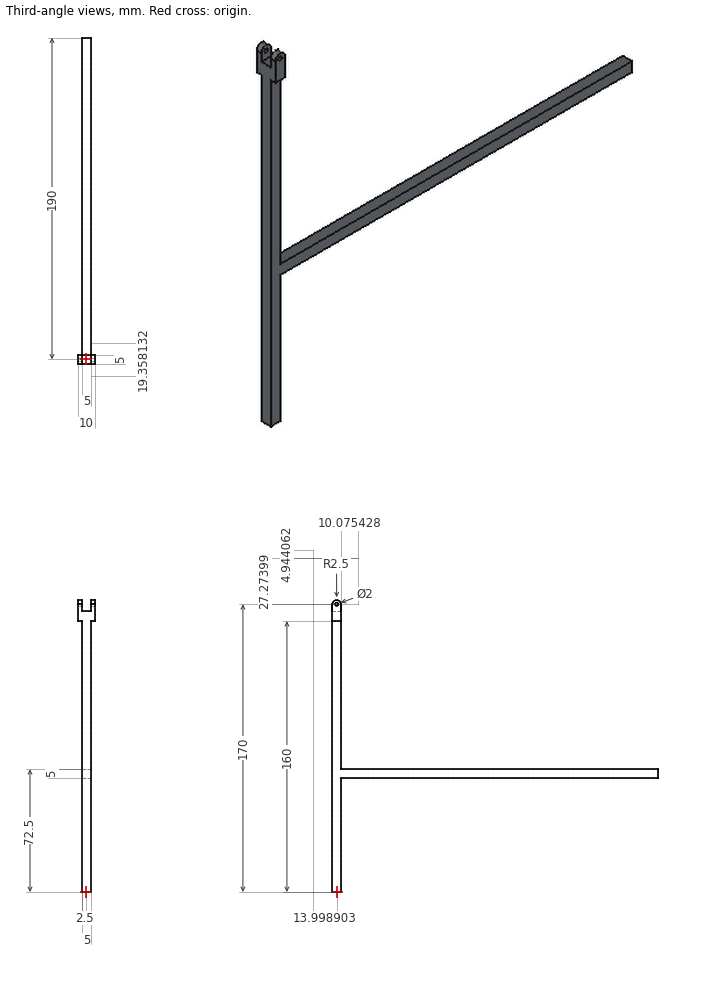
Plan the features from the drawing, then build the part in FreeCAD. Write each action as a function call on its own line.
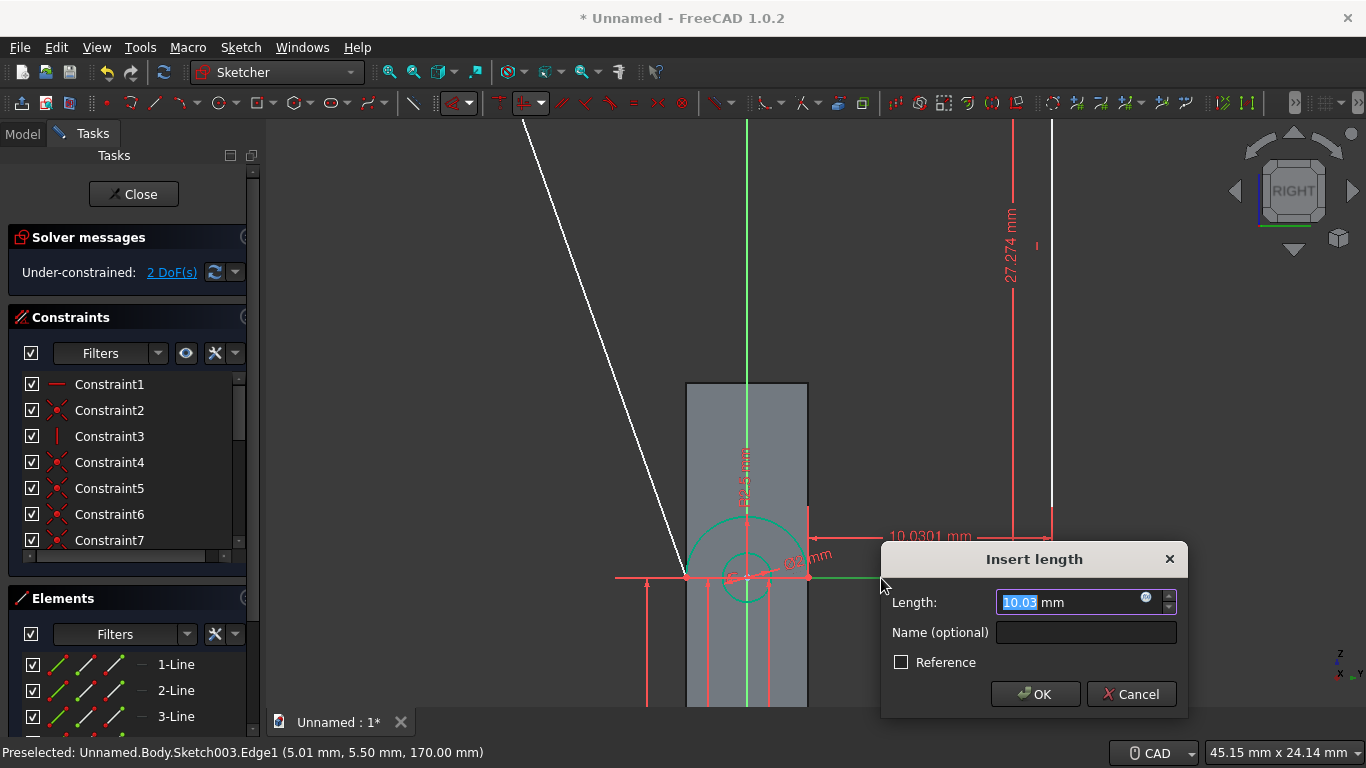
text(10.075428)
key(Return)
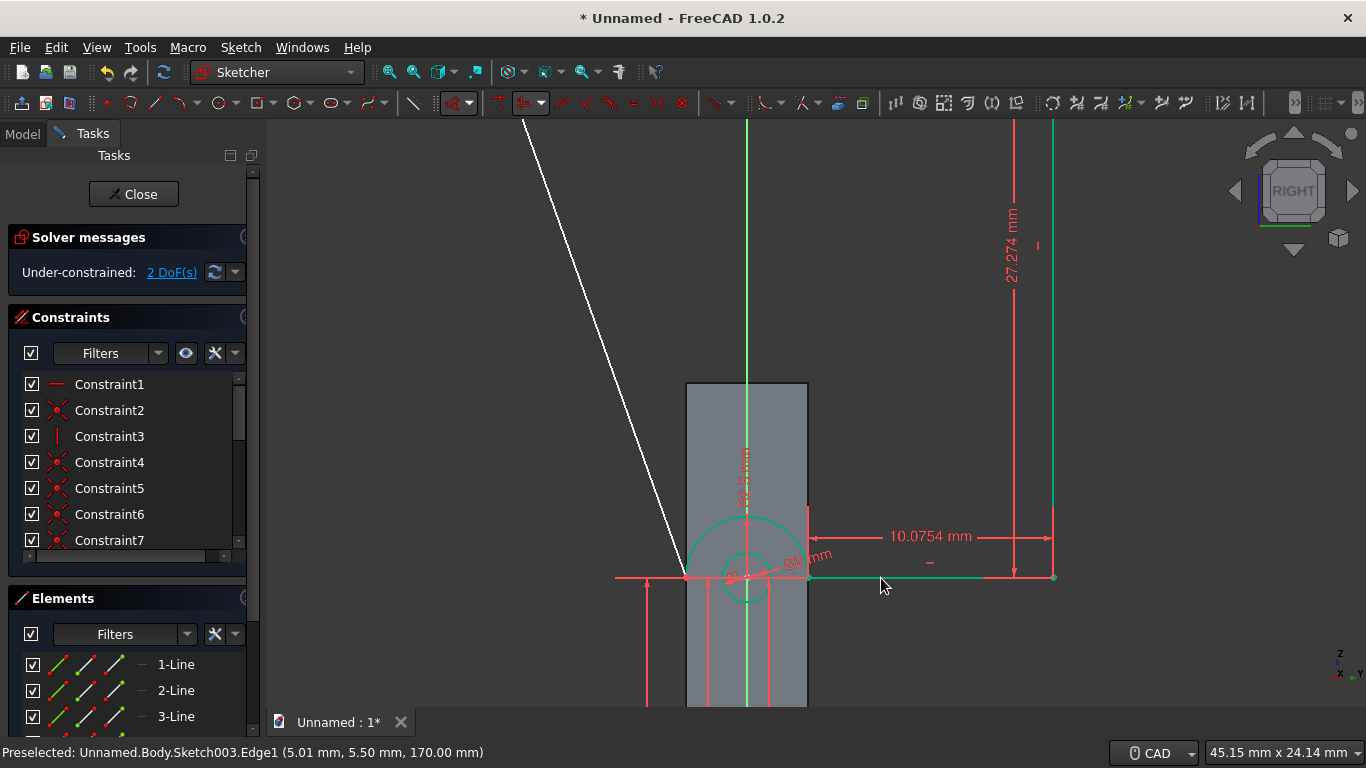
scroll(762, 589, down, 4)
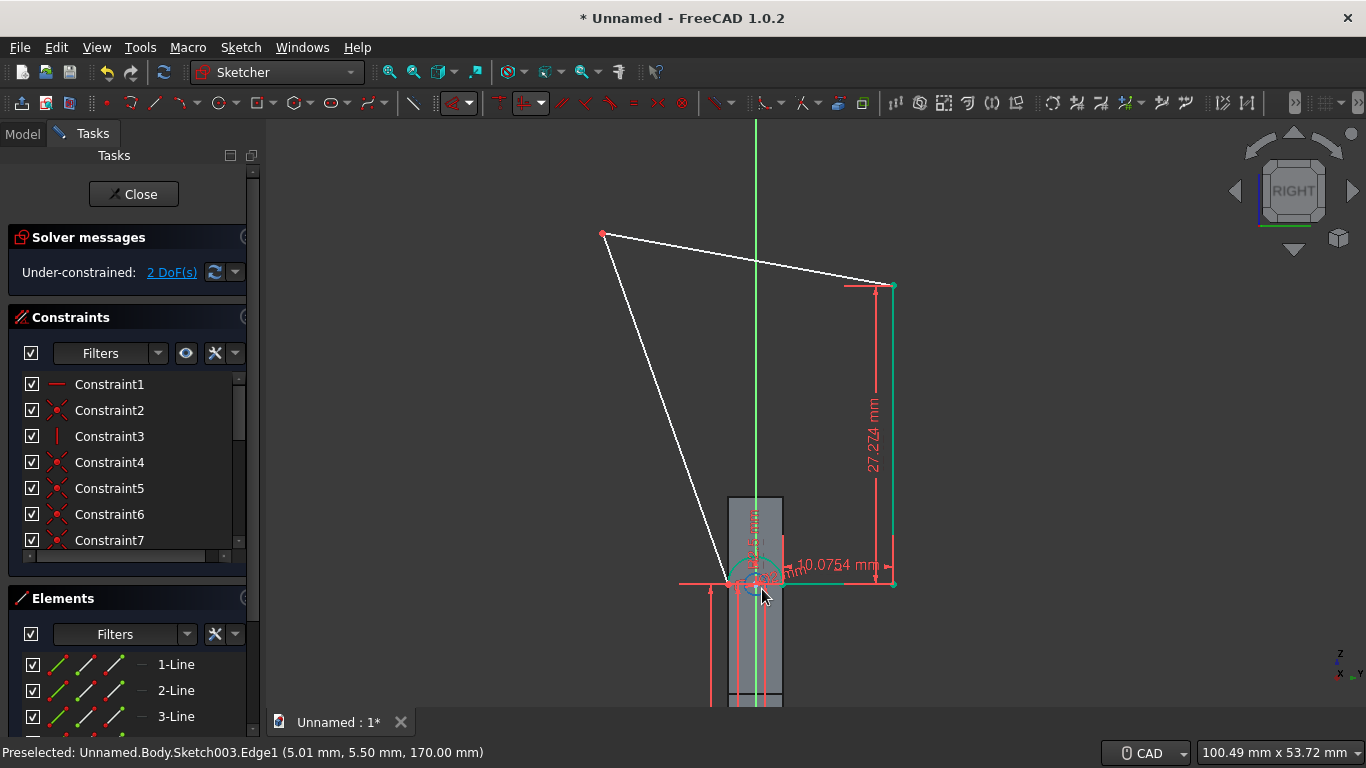
click(806, 270)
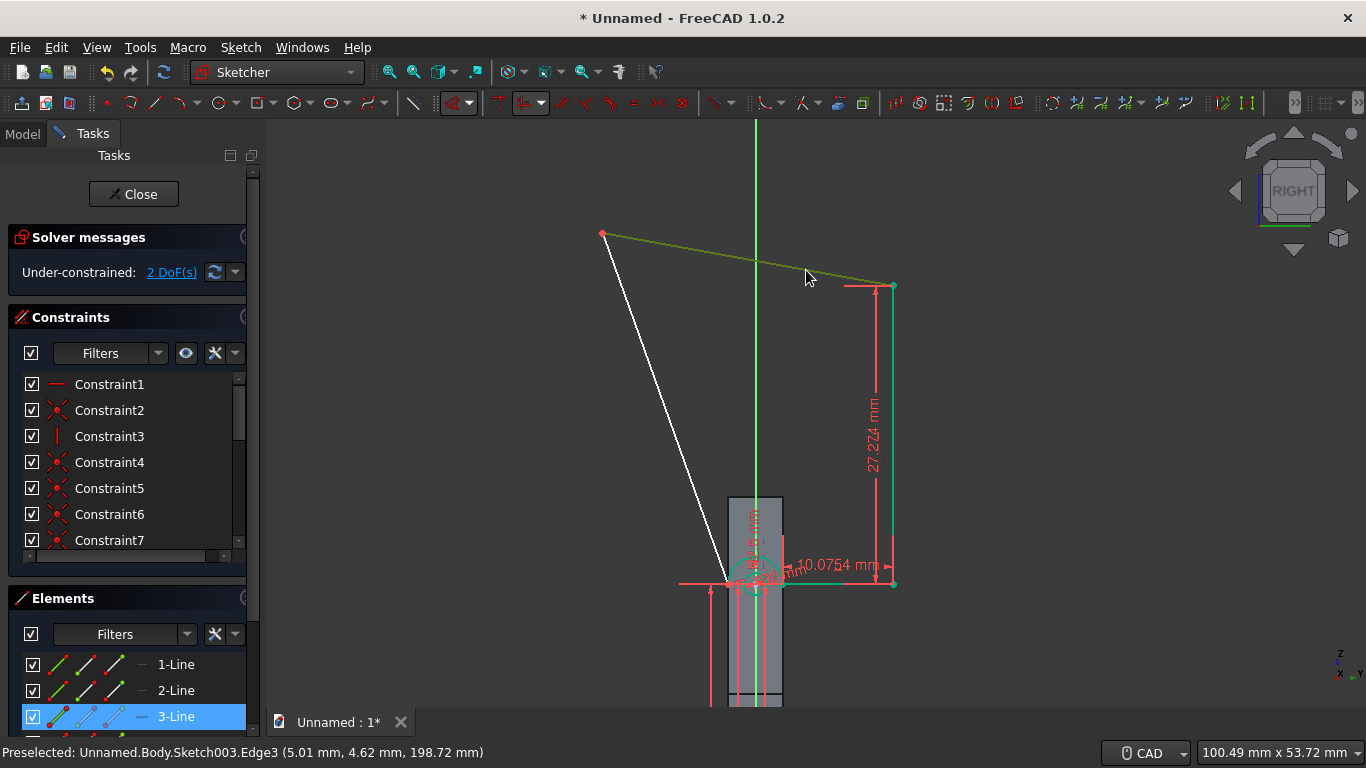
click(472, 104)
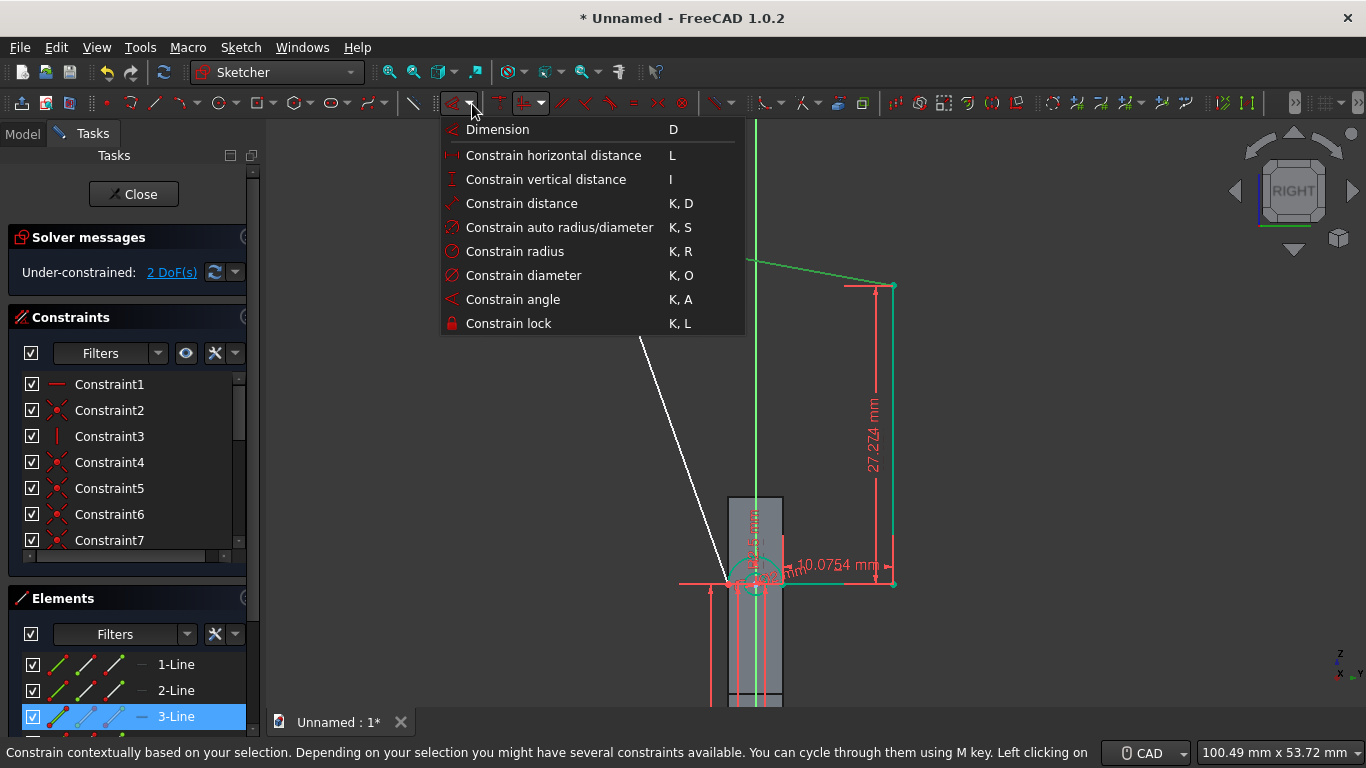
click(593, 179)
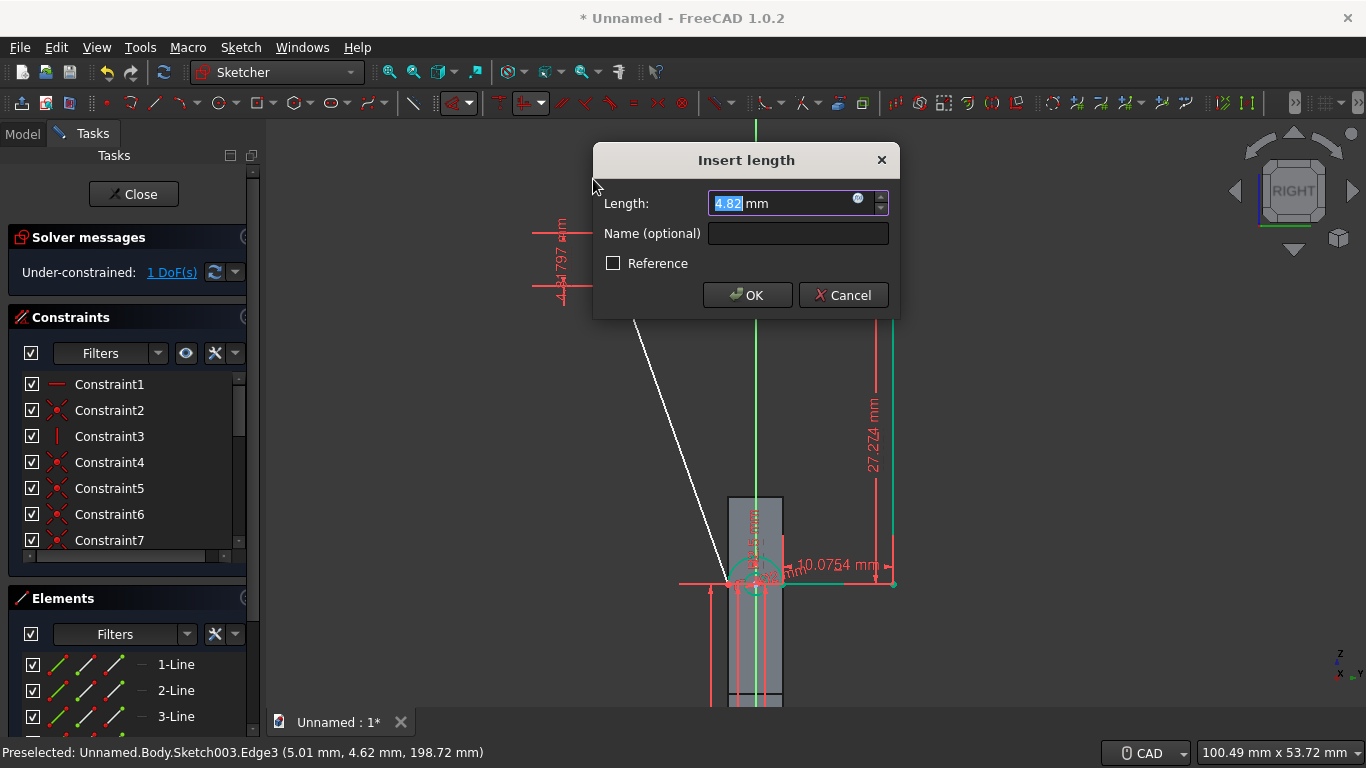
text(4.944062)
key(Return)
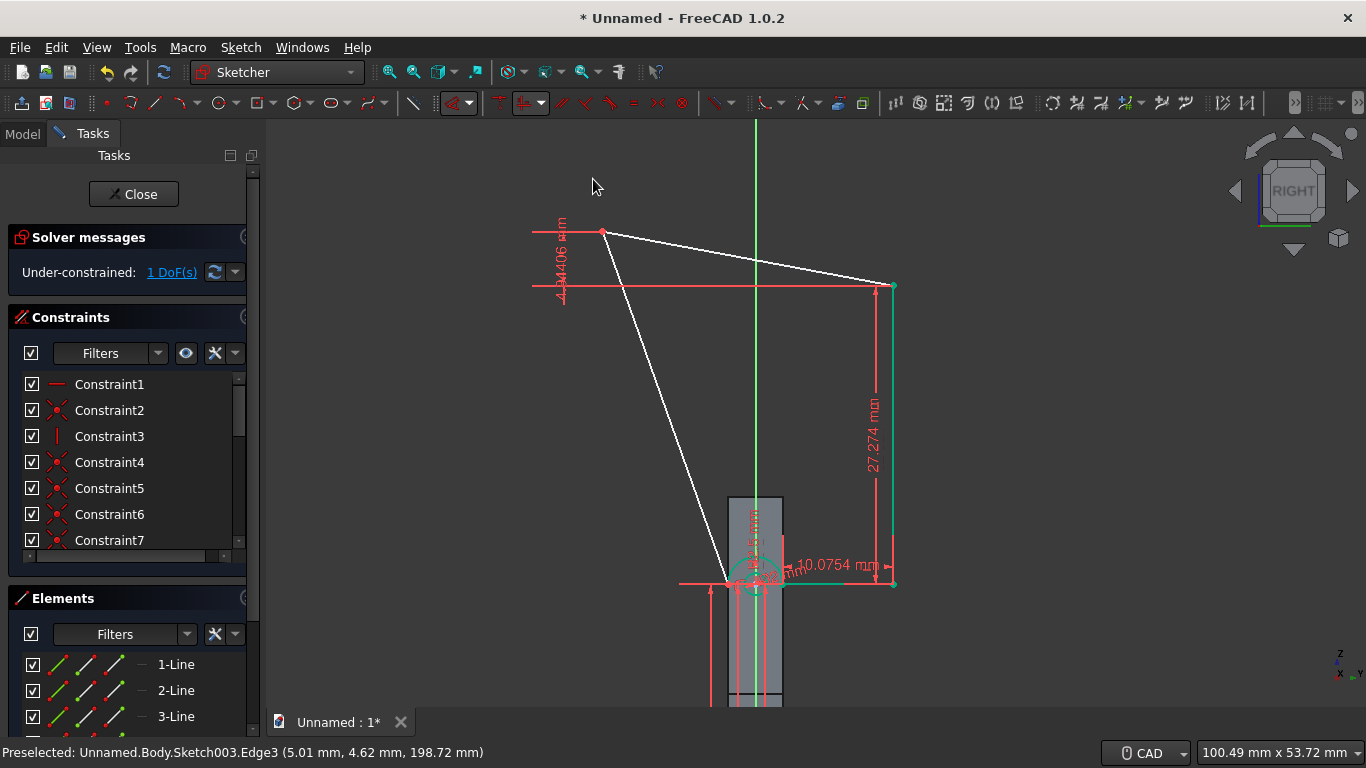
click(603, 232)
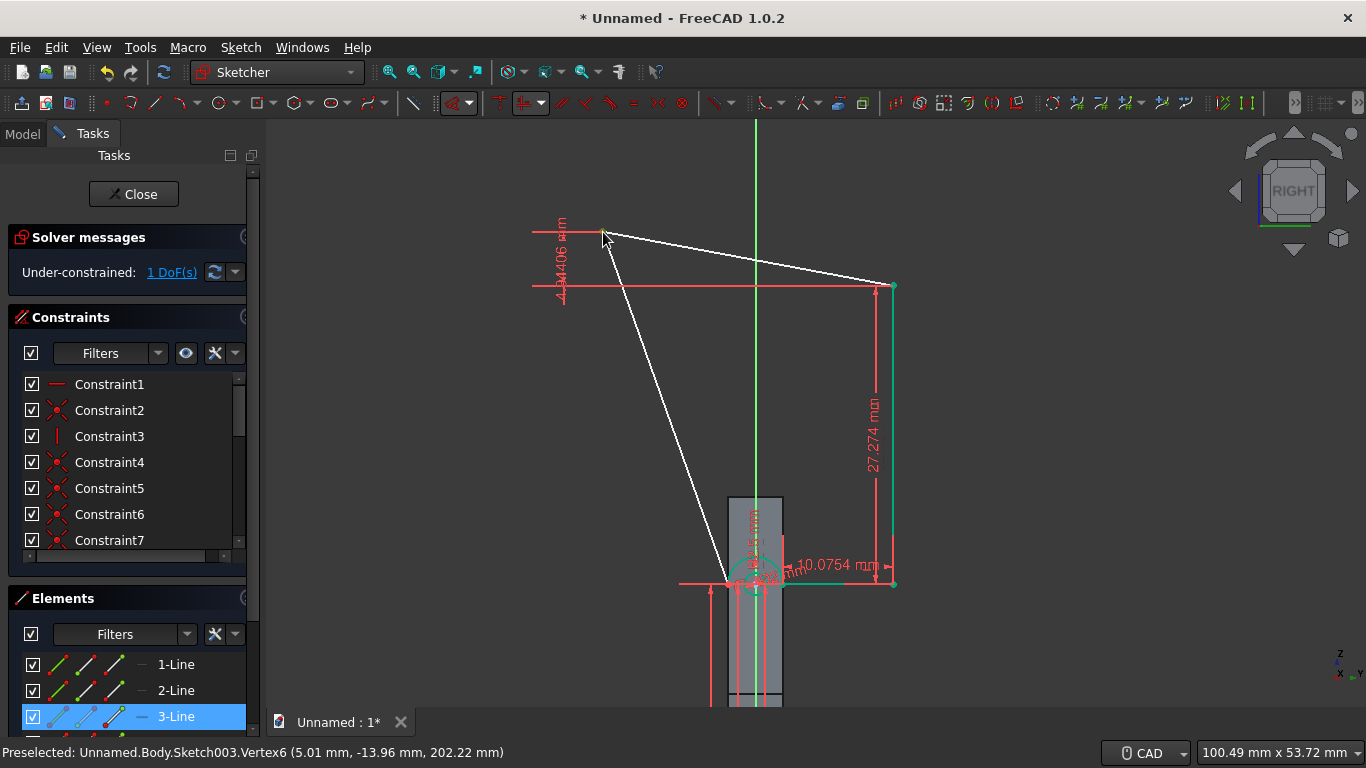
click(472, 104)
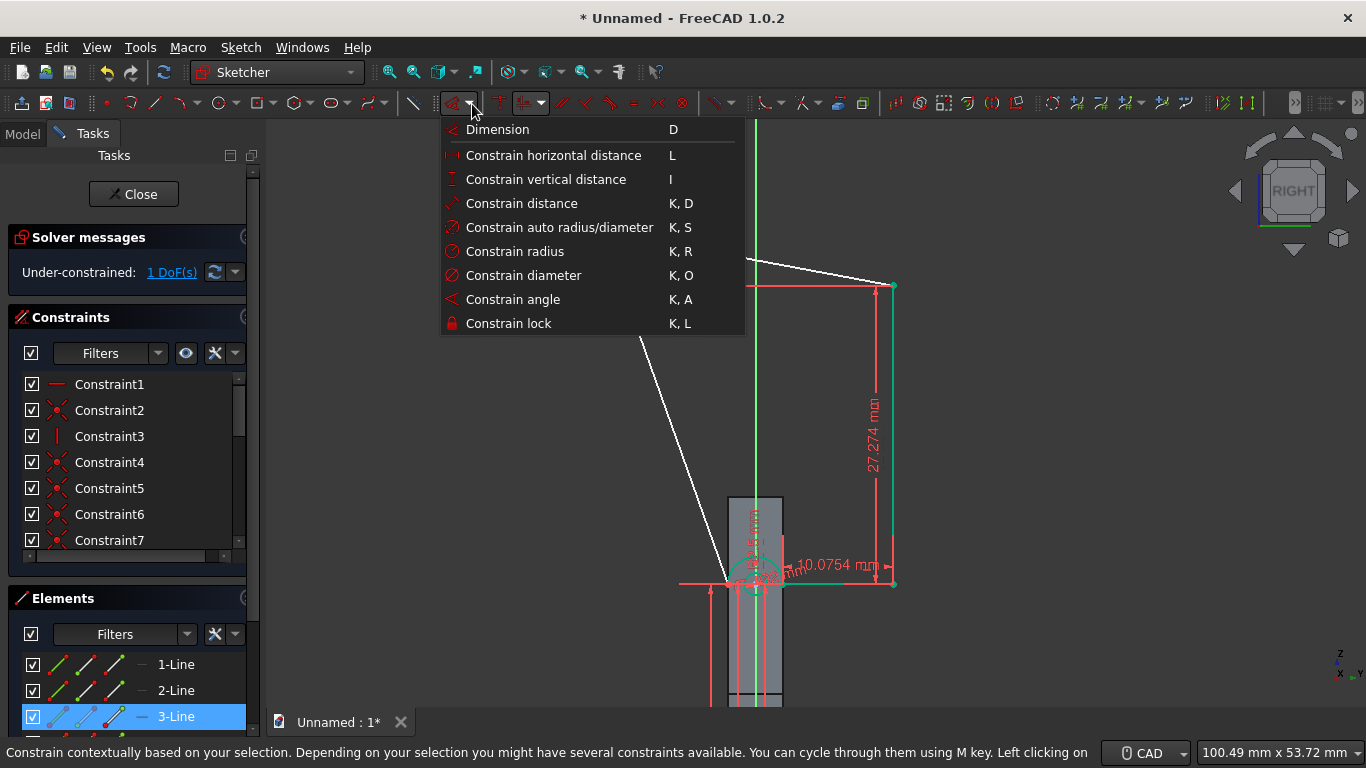
click(593, 155)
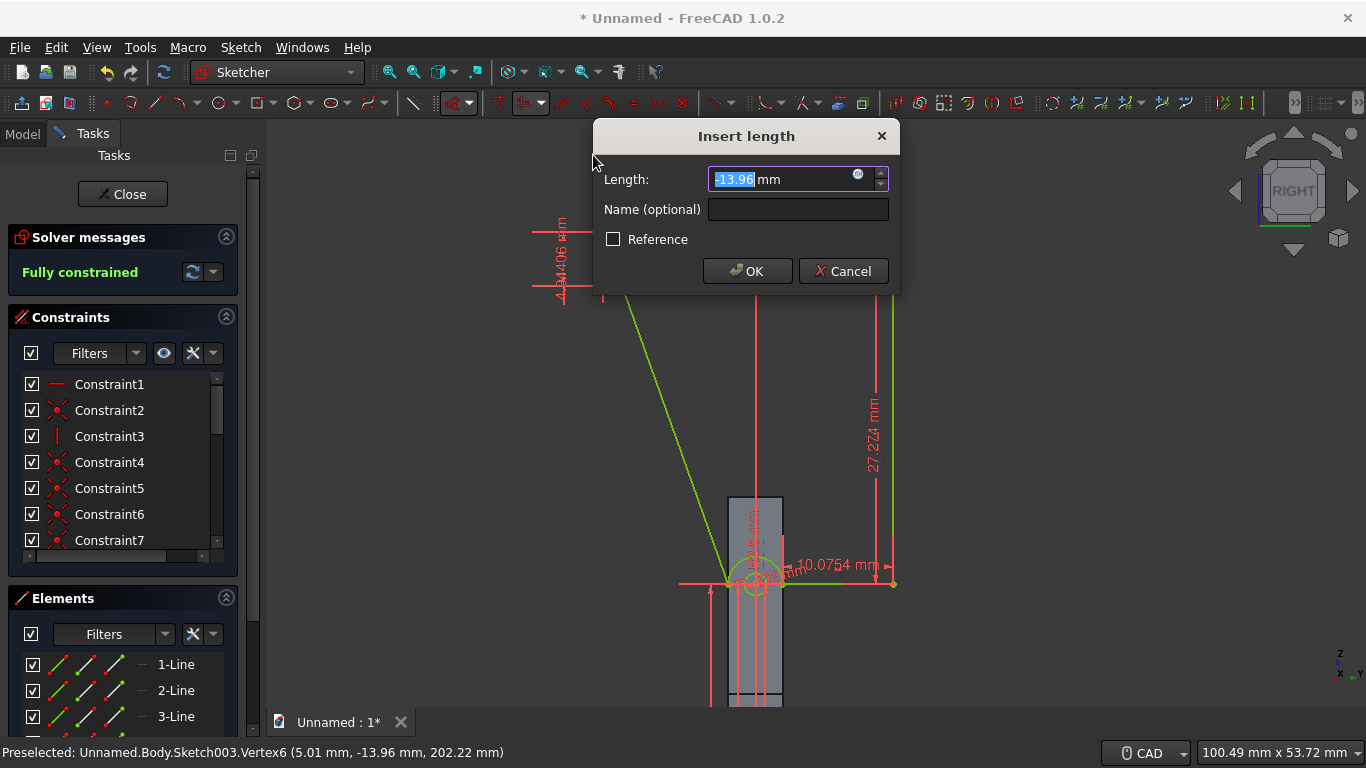
text(-13.998903)
key(Return)